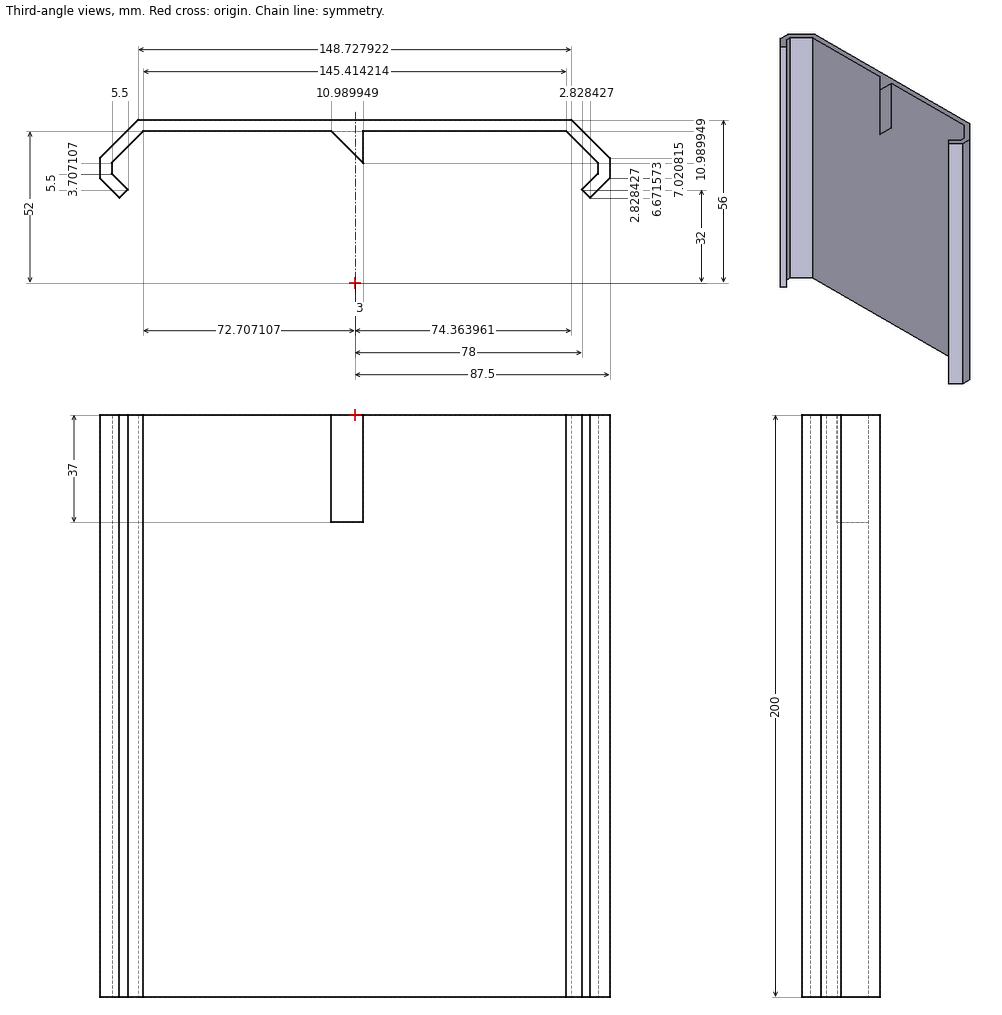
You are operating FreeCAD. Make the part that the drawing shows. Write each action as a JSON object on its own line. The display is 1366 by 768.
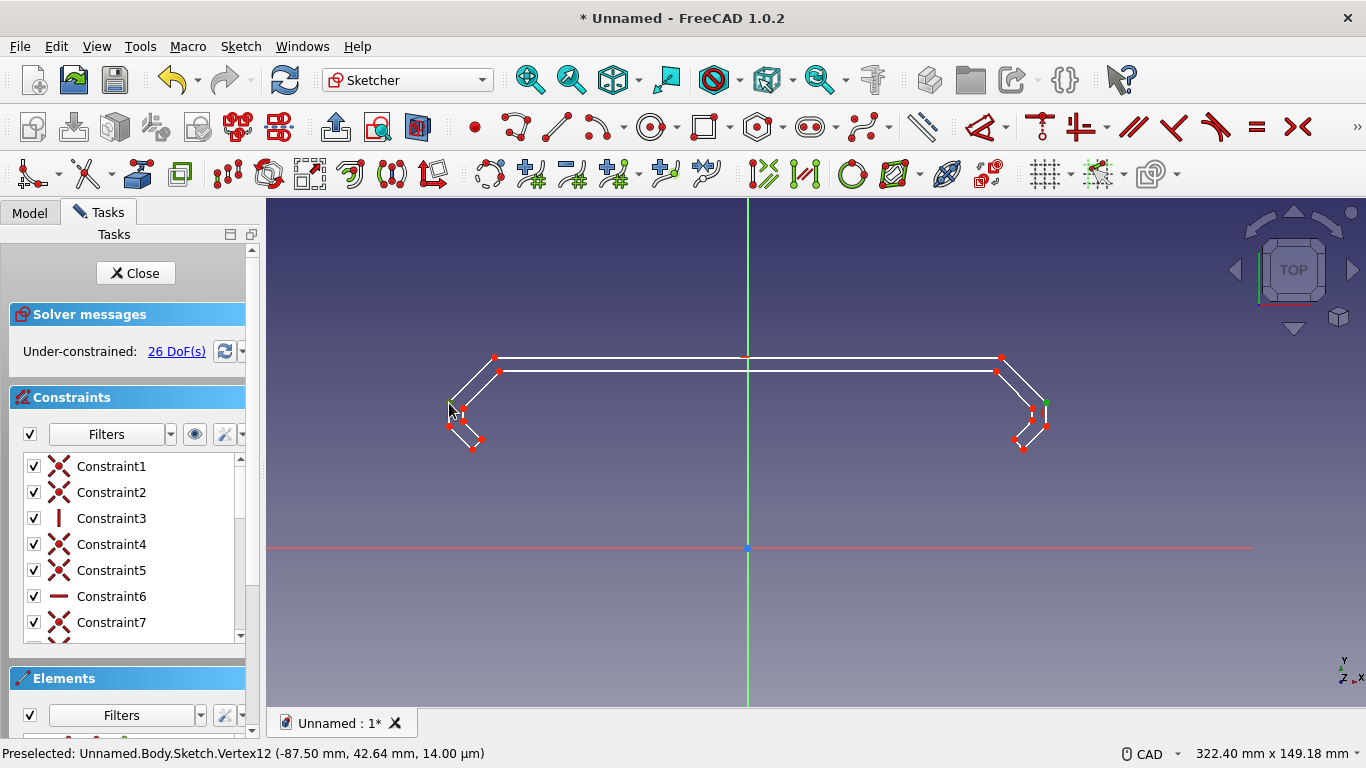
{"action": "left_click", "coordinate": [748, 647]}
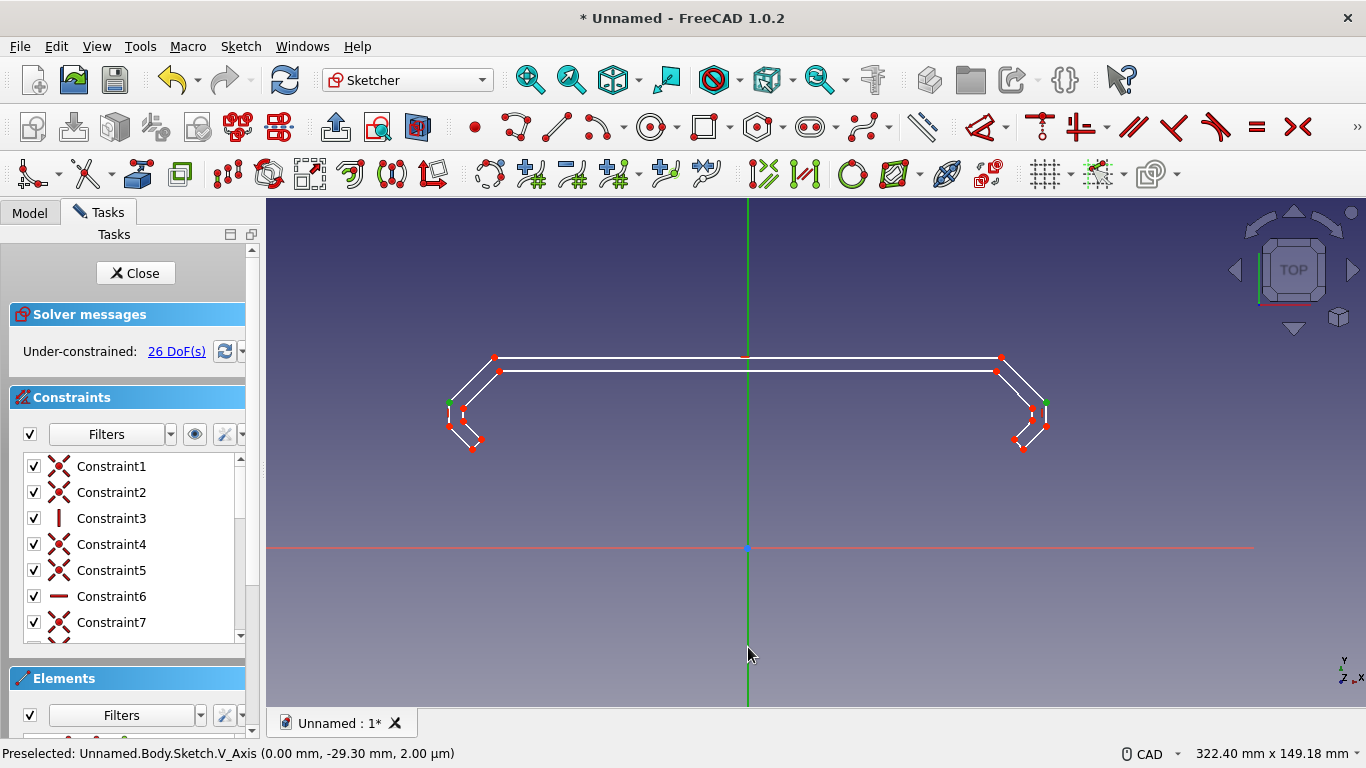
{"action": "left_click", "coordinate": [1298, 128]}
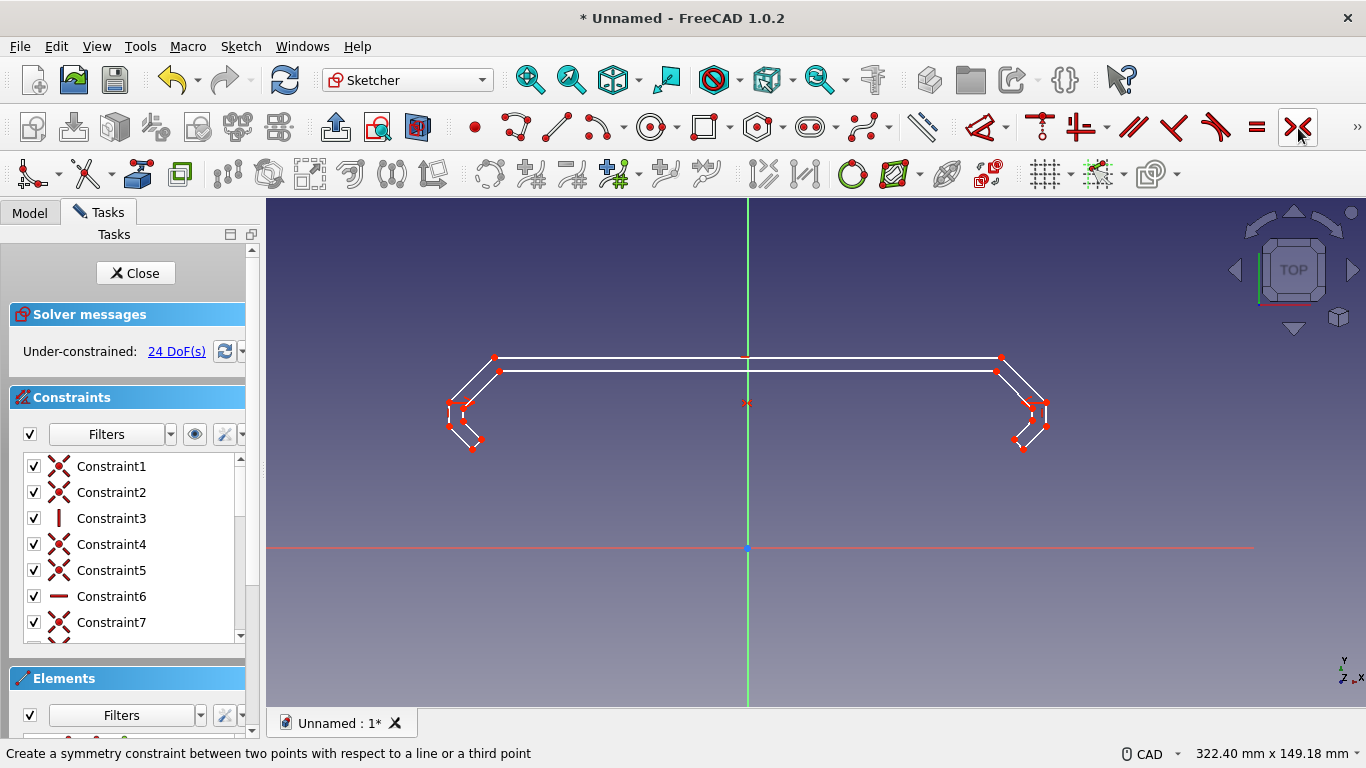
{"action": "left_click", "coordinate": [1023, 450]}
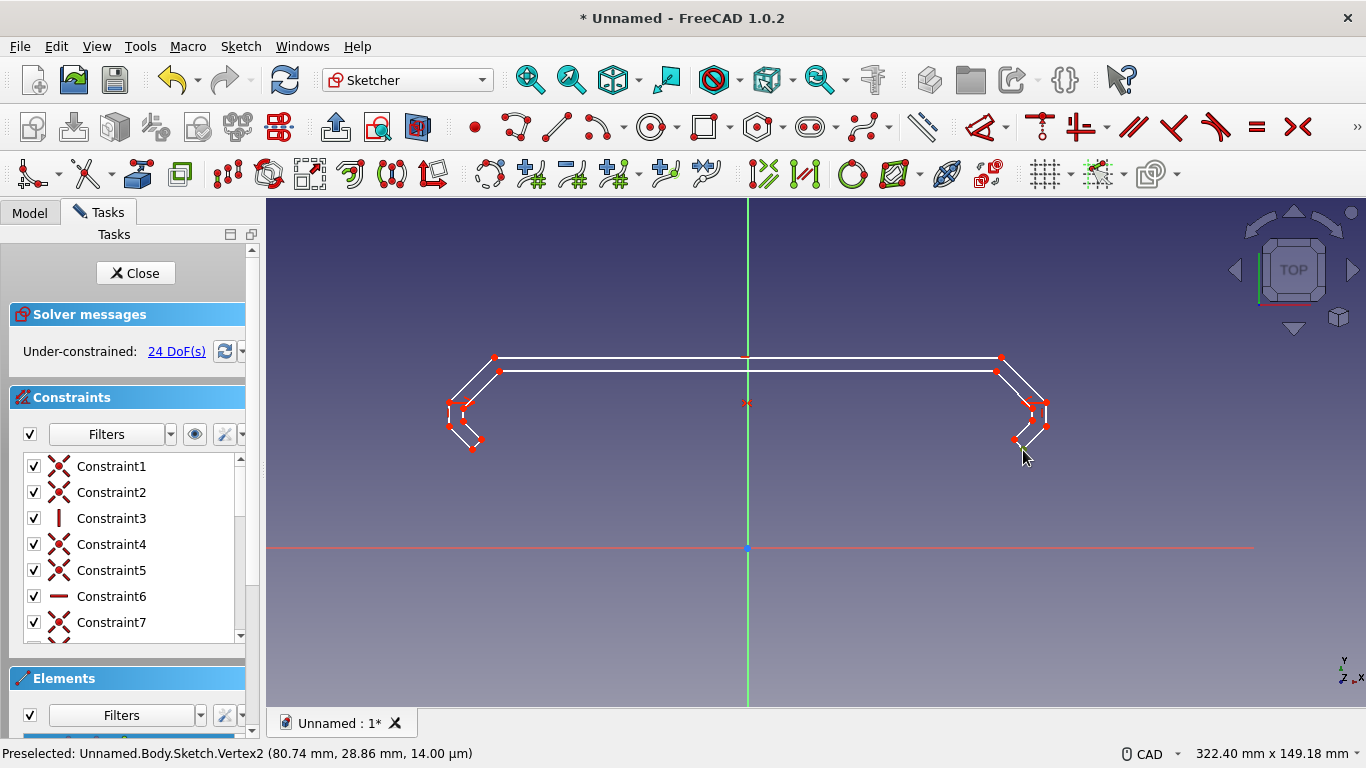
{"action": "left_click", "coordinate": [472, 450]}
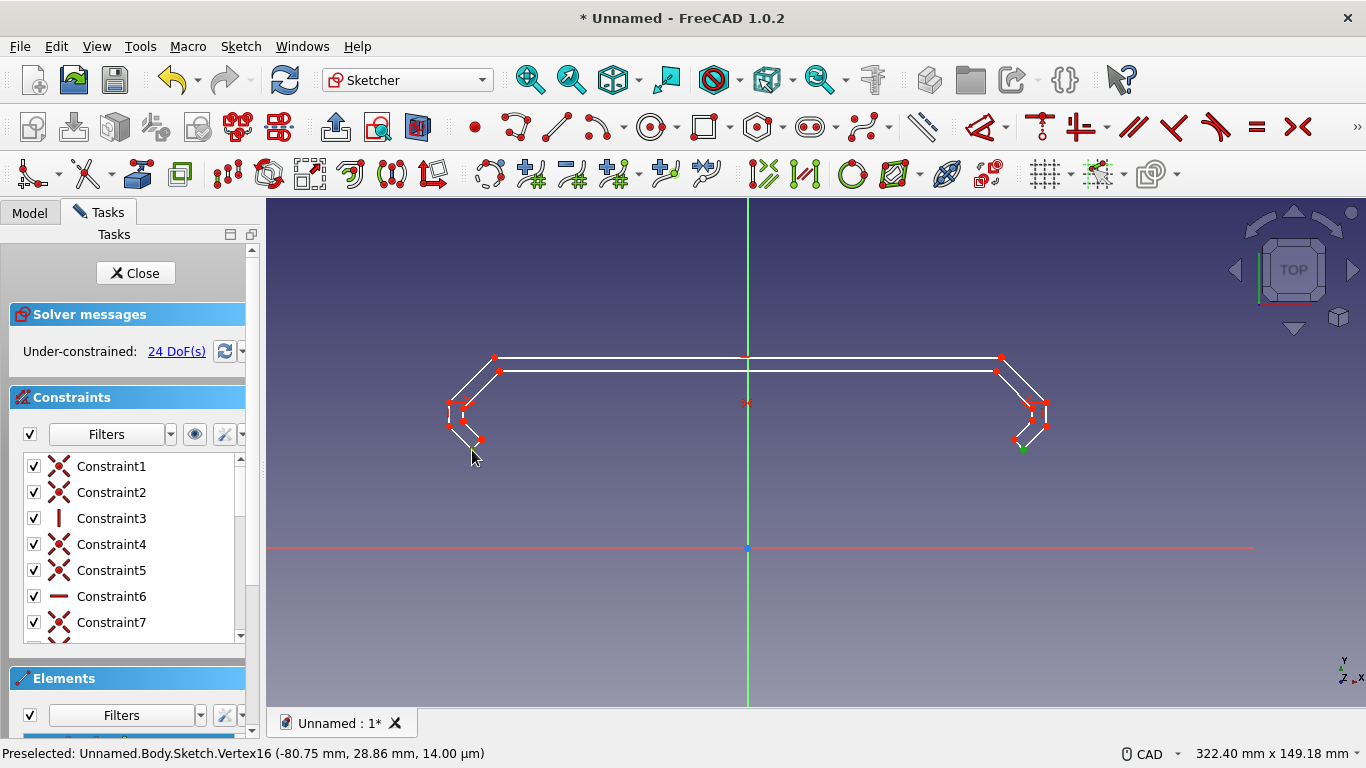
{"action": "left_click", "coordinate": [748, 647]}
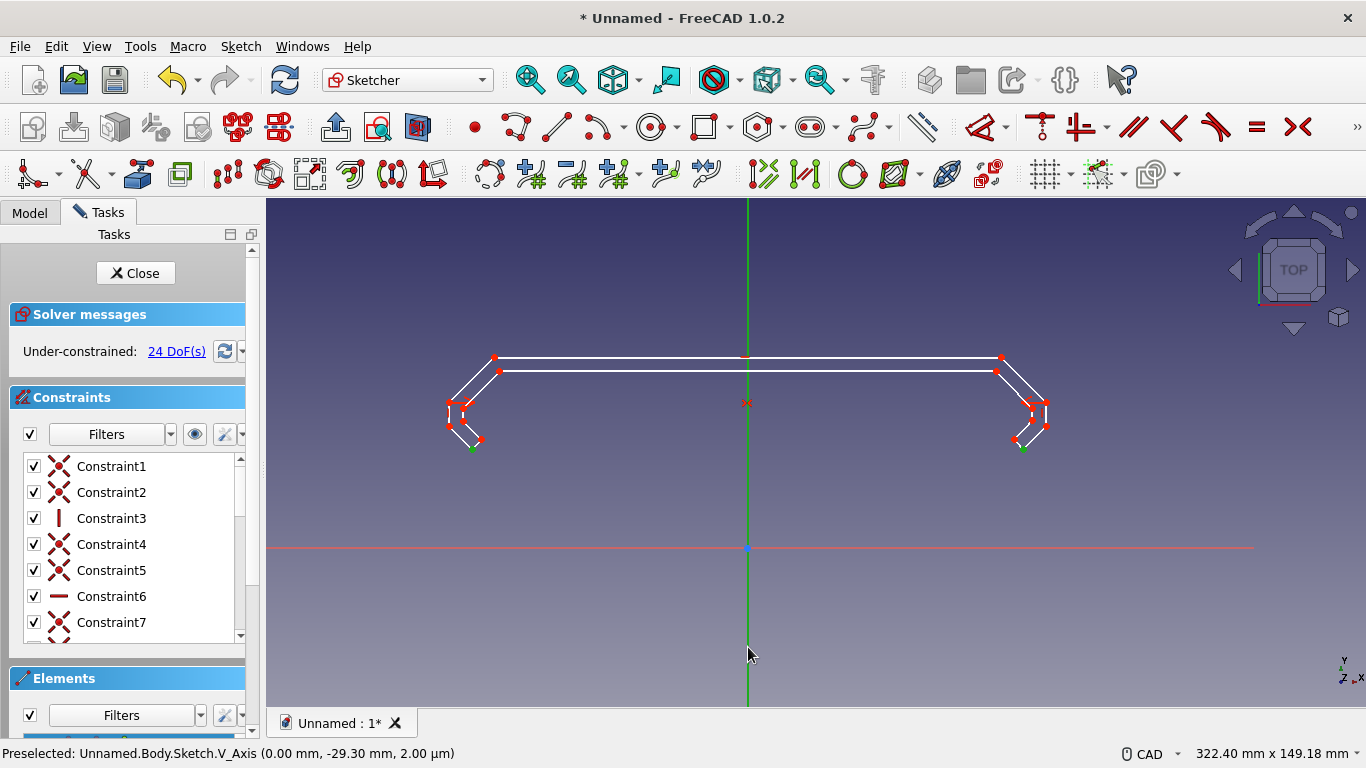
{"action": "left_click", "coordinate": [1298, 128]}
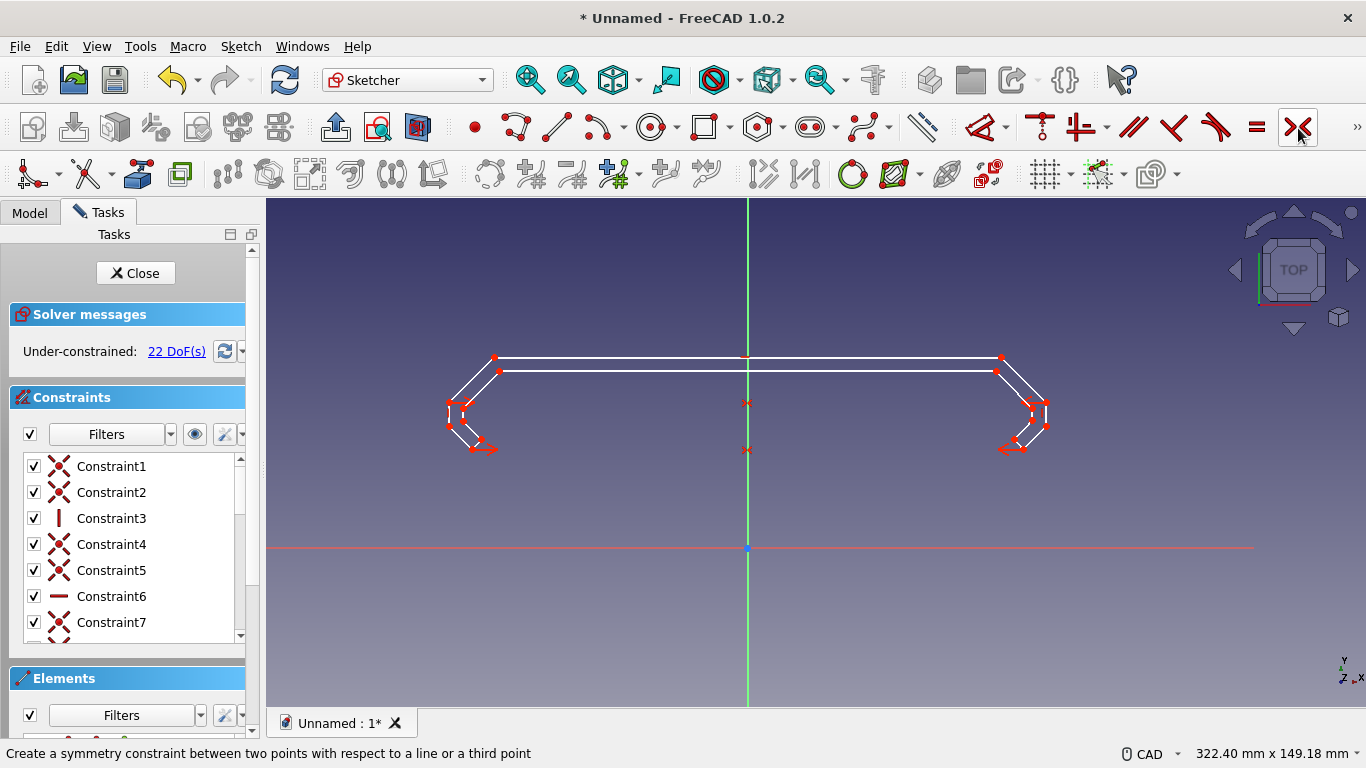
{"action": "left_click", "coordinate": [1014, 440]}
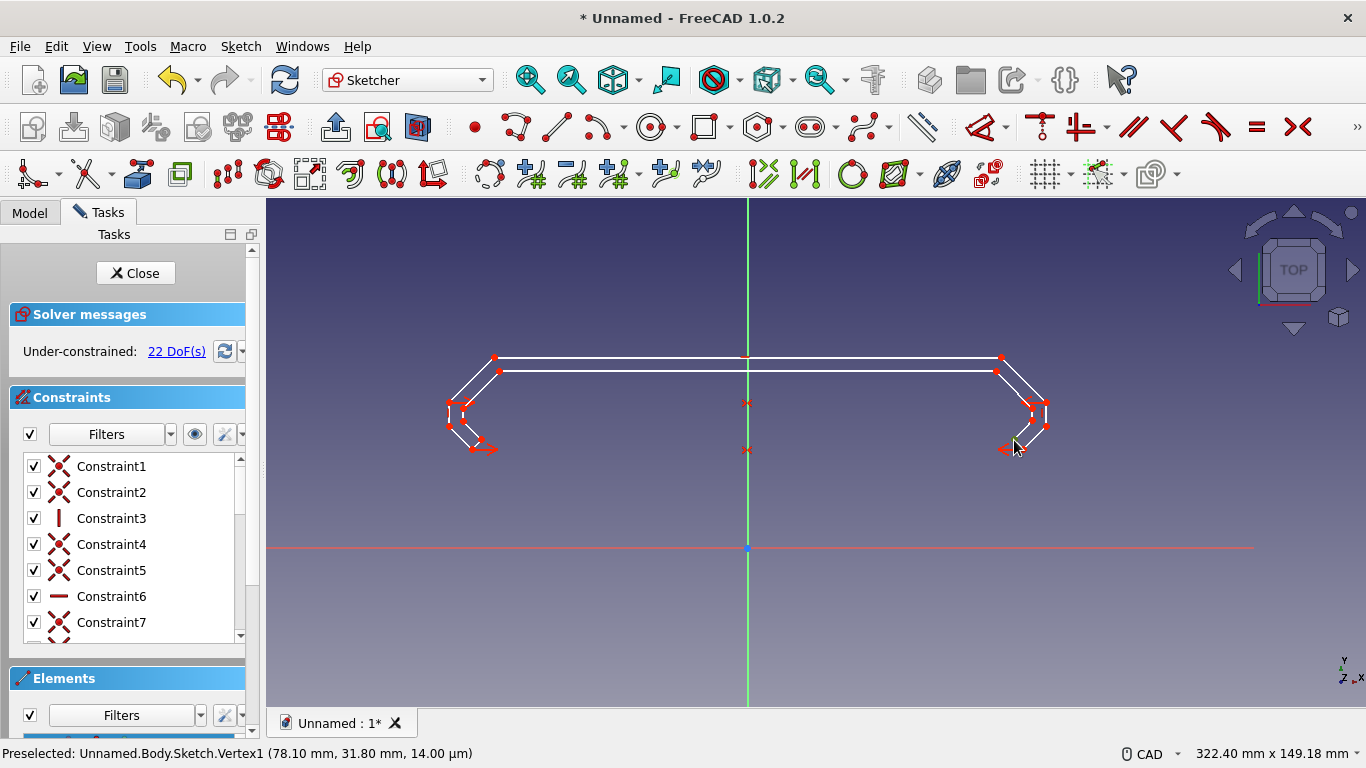
{"action": "left_click", "coordinate": [481, 440]}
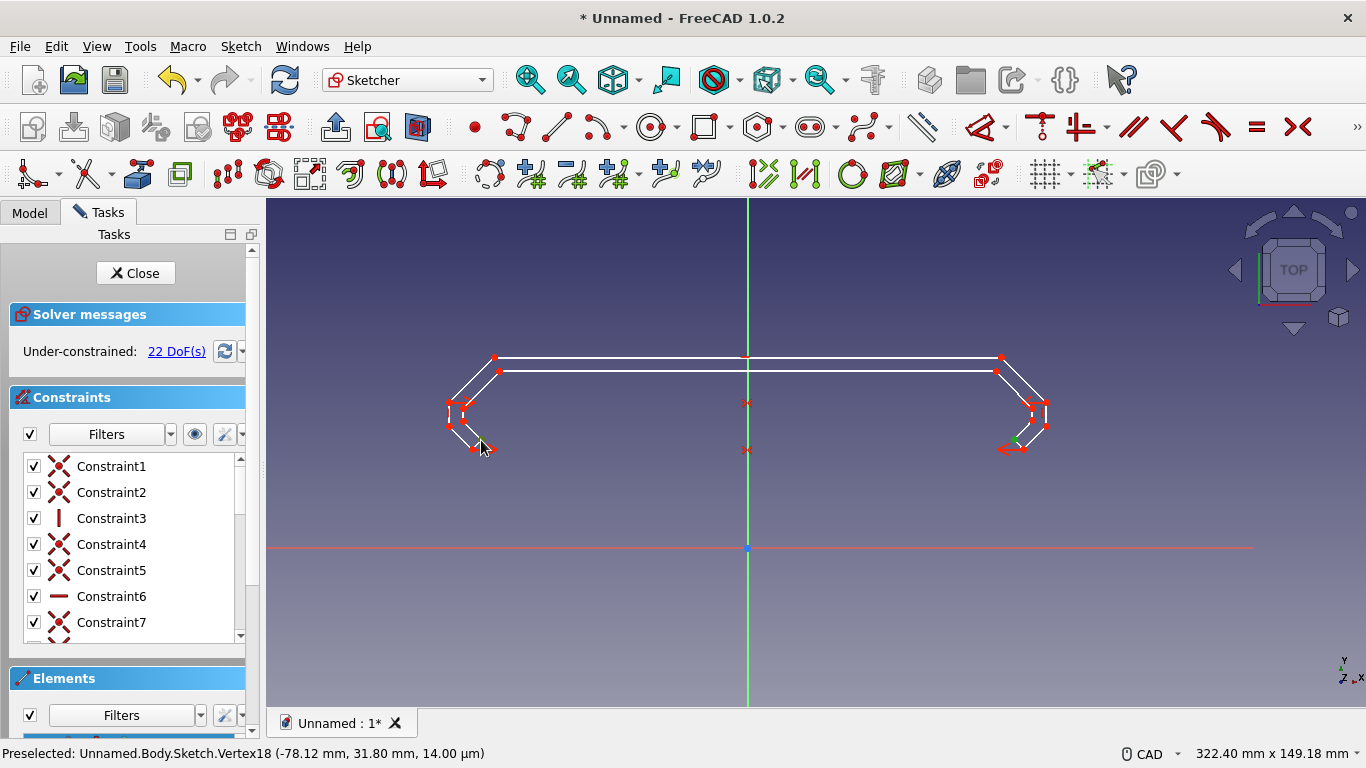
{"action": "left_click", "coordinate": [748, 647]}